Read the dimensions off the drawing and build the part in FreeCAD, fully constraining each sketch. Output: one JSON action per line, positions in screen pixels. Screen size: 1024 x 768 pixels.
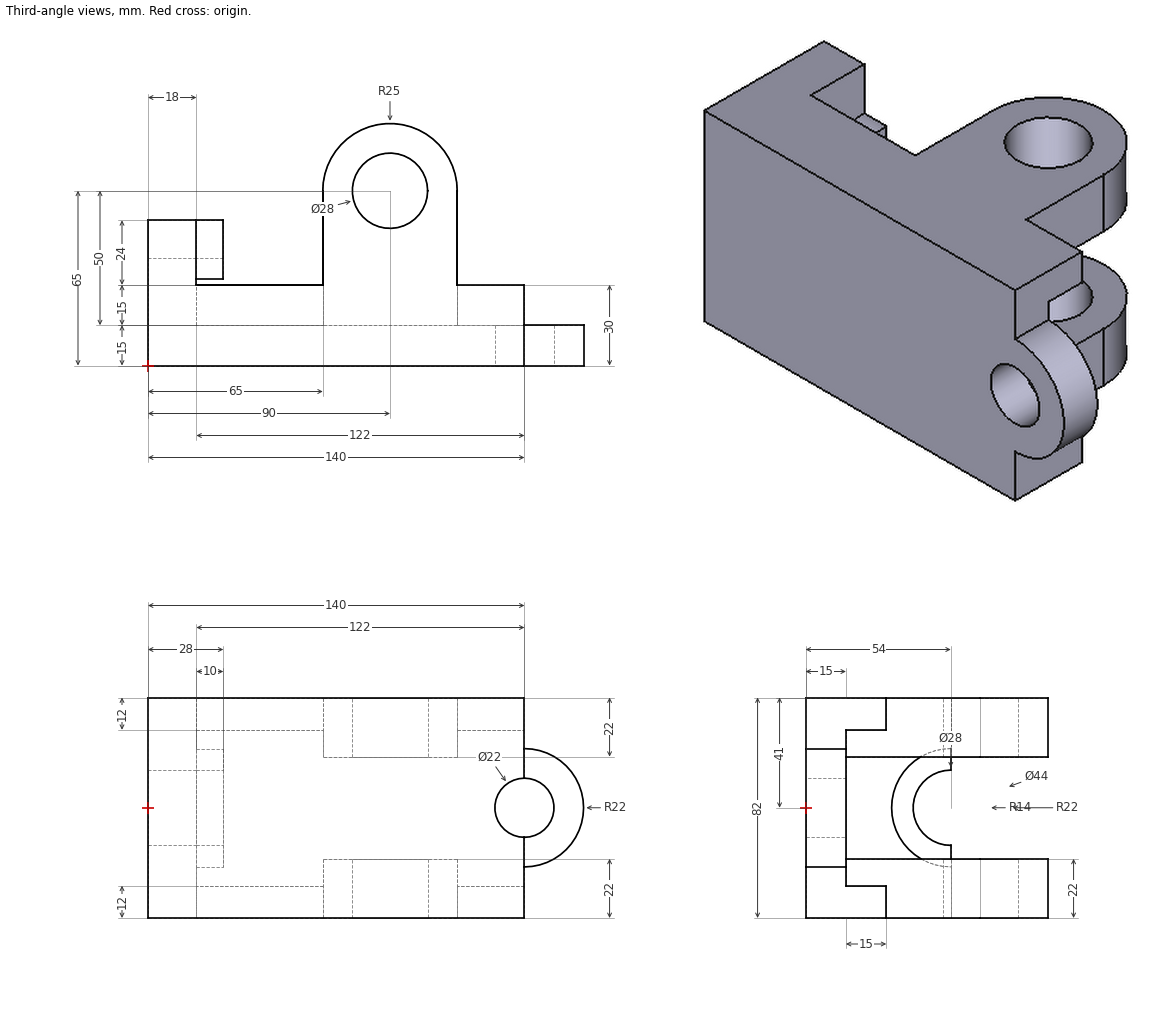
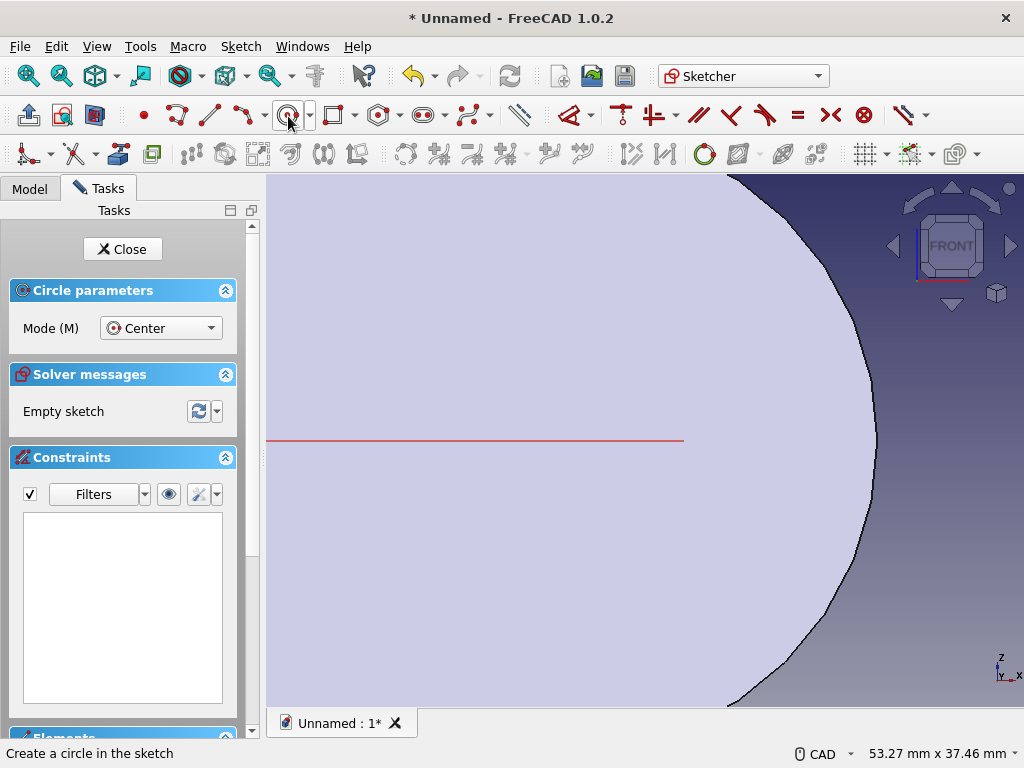
{"action": "left_click", "coordinate": [564, 440]}
{"action": "left_click", "coordinate": [675, 330]}
{"action": "key", "text": "Escape"}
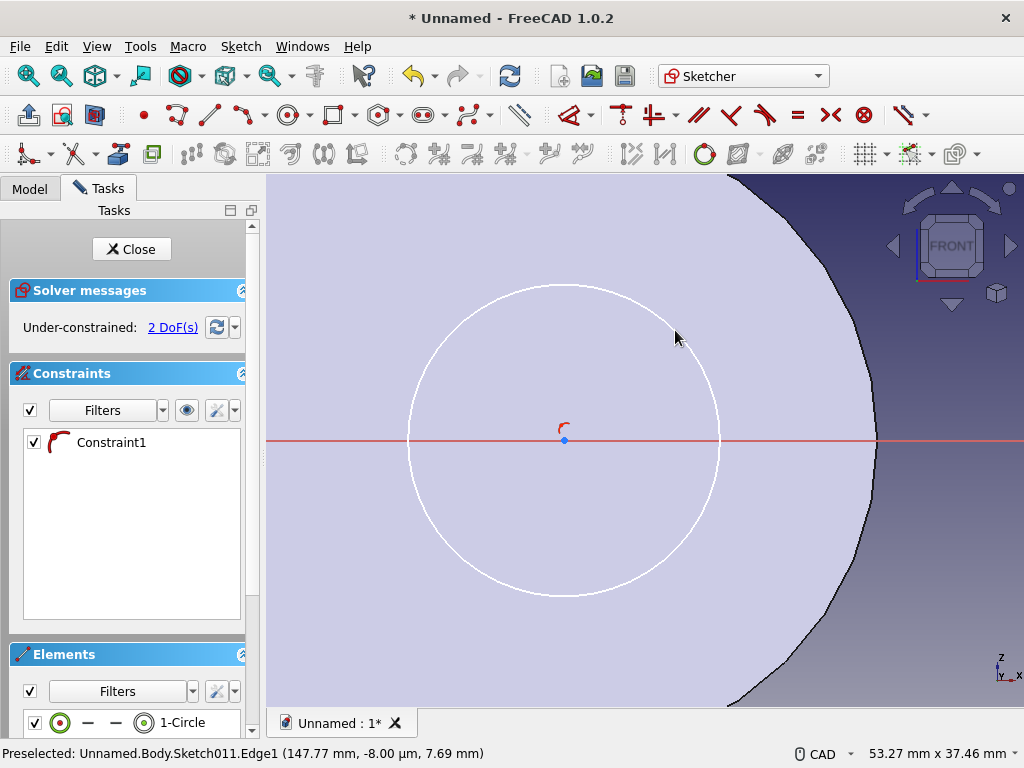
{"action": "key", "text": "d"}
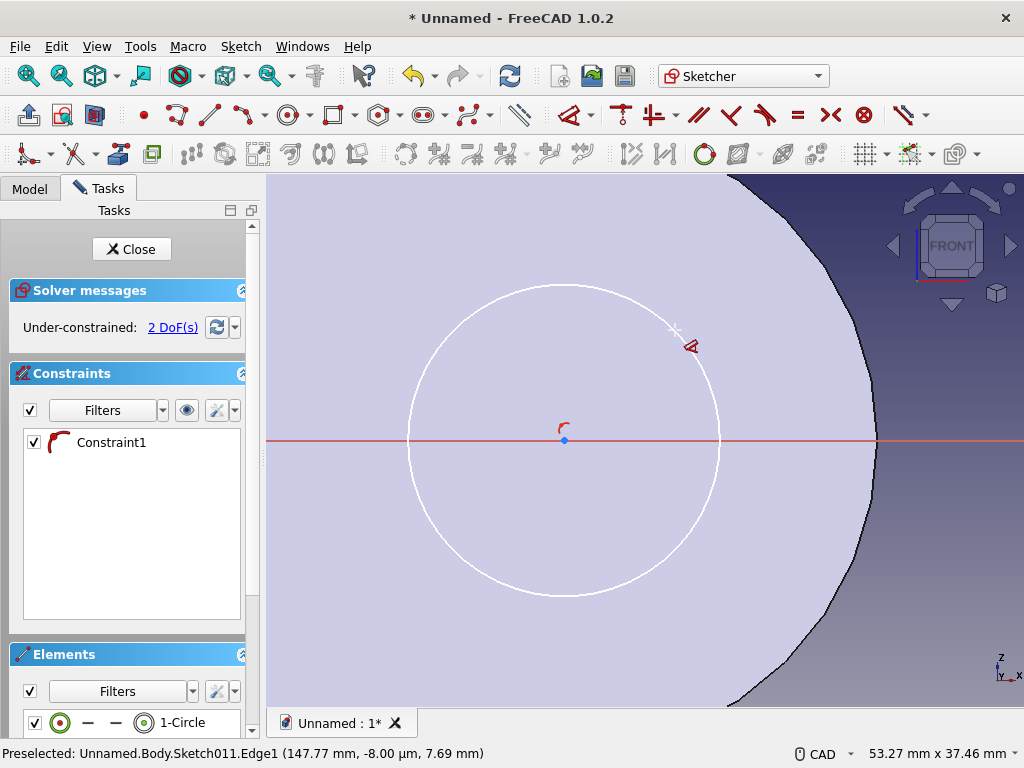
{"action": "left_click", "coordinate": [674, 330]}
{"action": "left_click", "coordinate": [697, 307]}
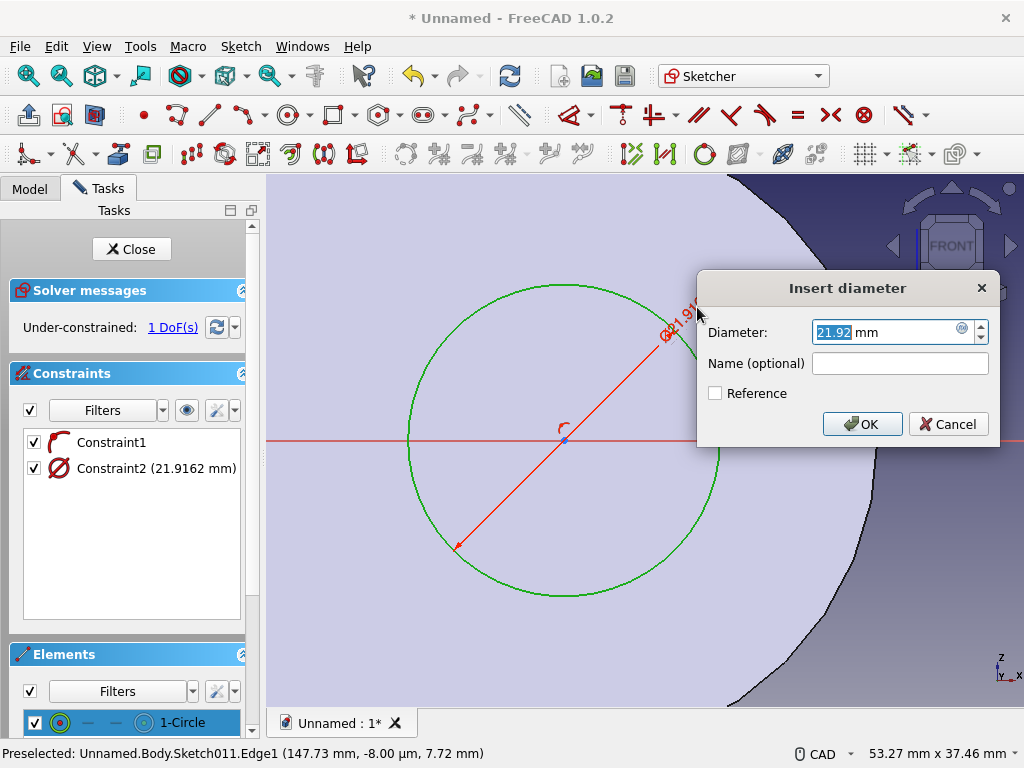
{"action": "type", "text": "22"}
{"action": "key", "text": "Return"}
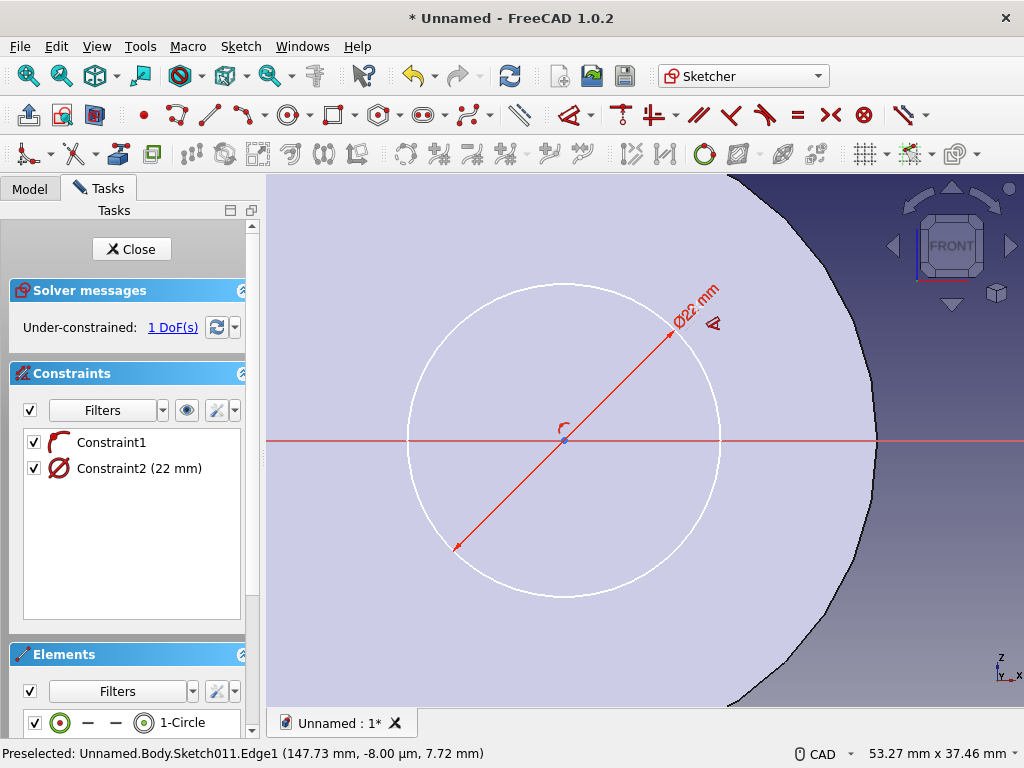
{"action": "left_click", "coordinate": [564, 440]}
{"action": "left_click", "coordinate": [429, 474]}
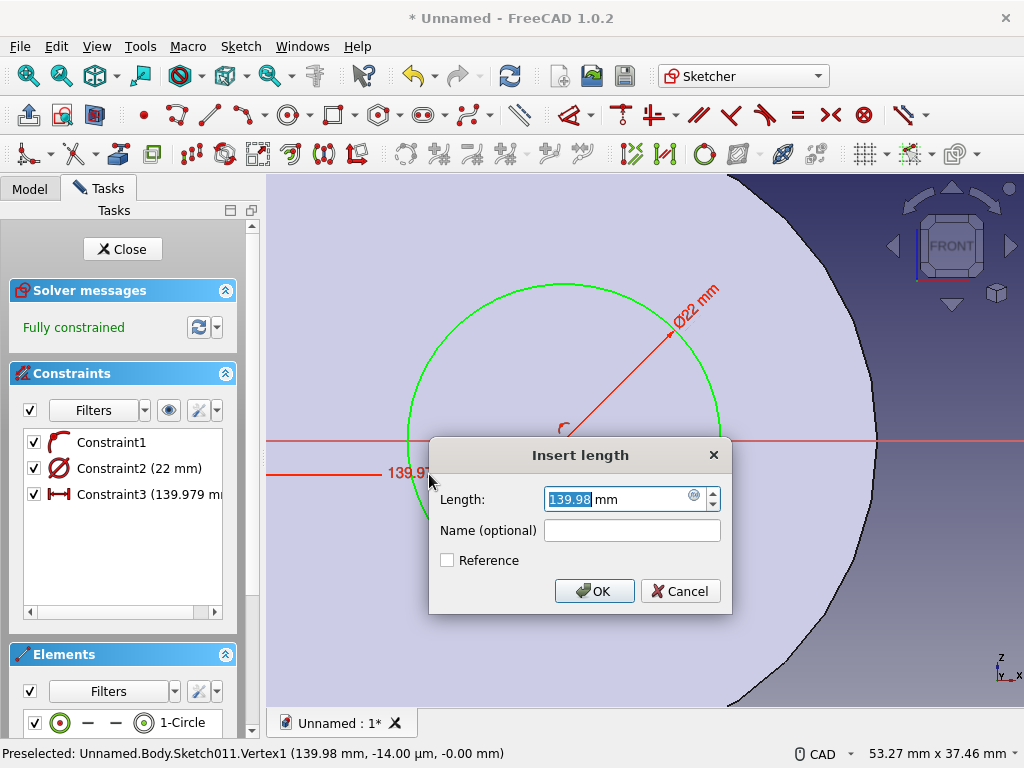
{"action": "type", "text": "140"}
{"action": "key", "text": "Return"}
{"action": "key", "text": "Escape"}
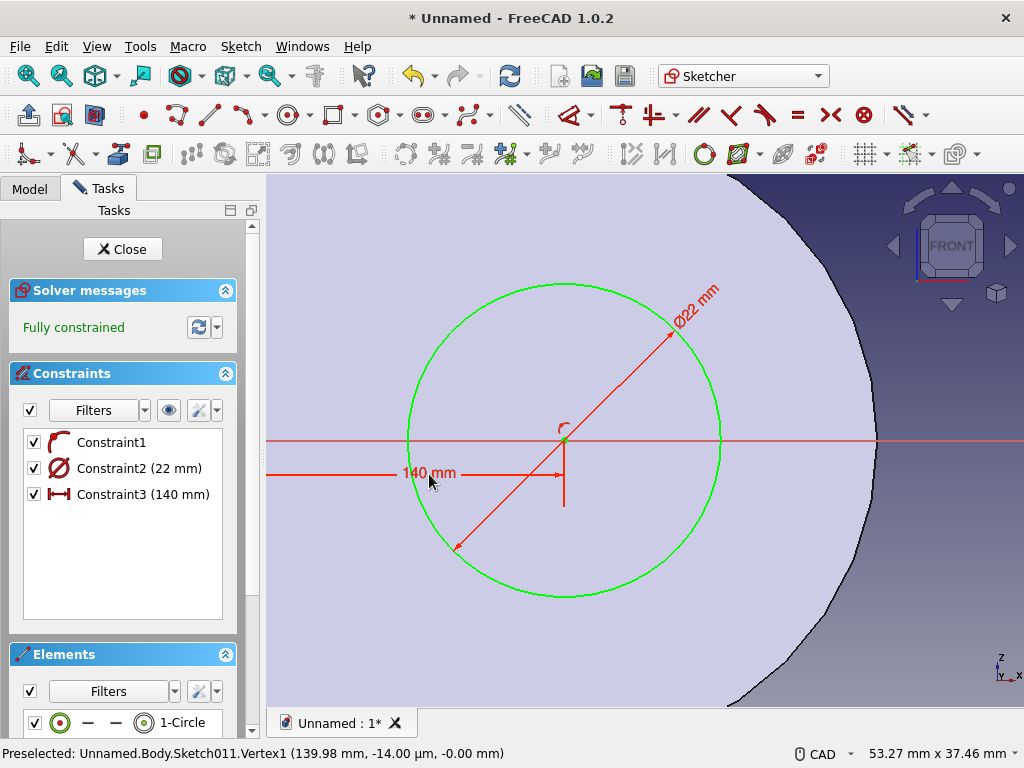
{"action": "left_click", "coordinate": [123, 249]}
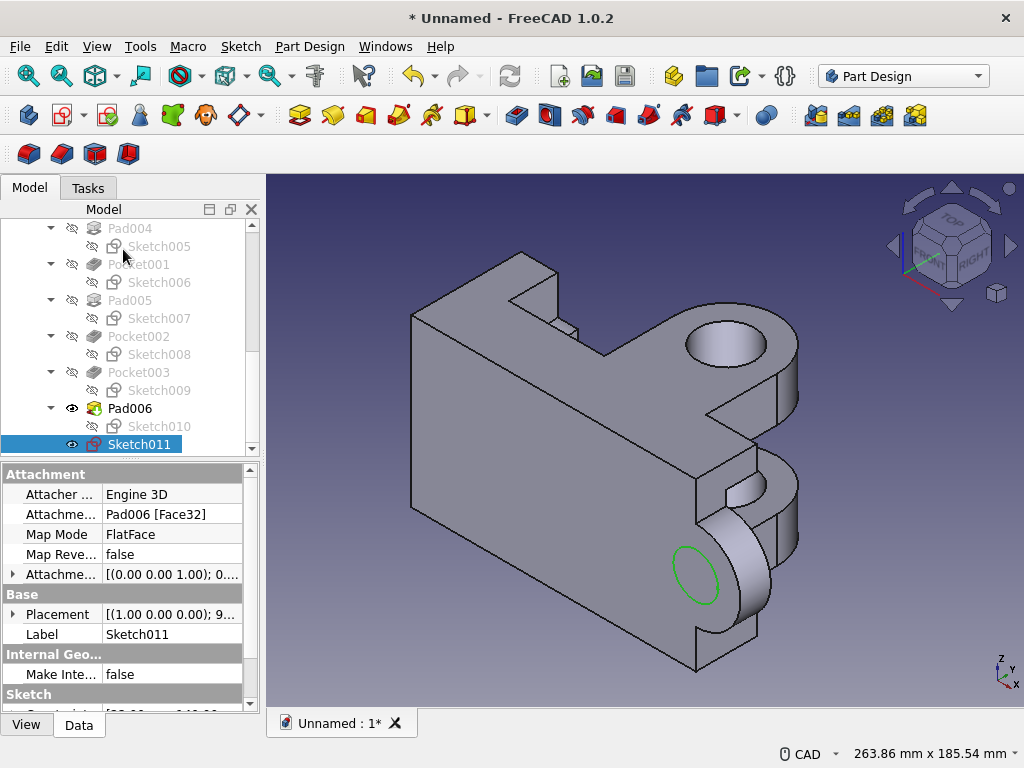
{"action": "left_click", "coordinate": [517, 116]}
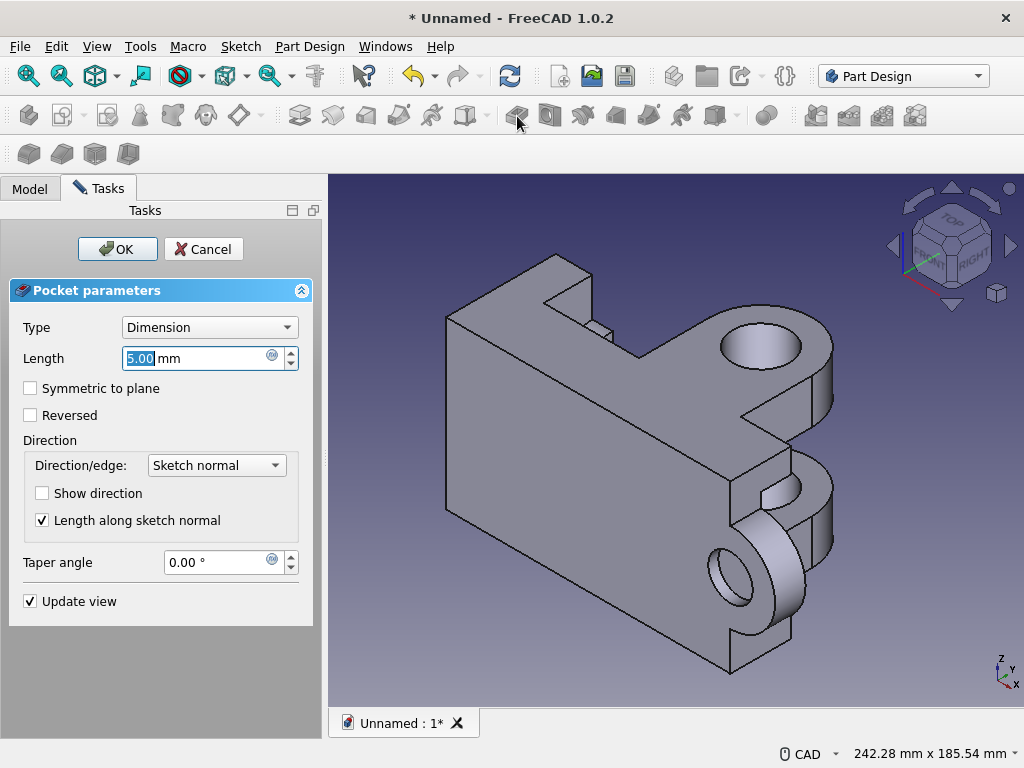
{"action": "type", "text": "15"}
{"action": "key", "text": "Tab"}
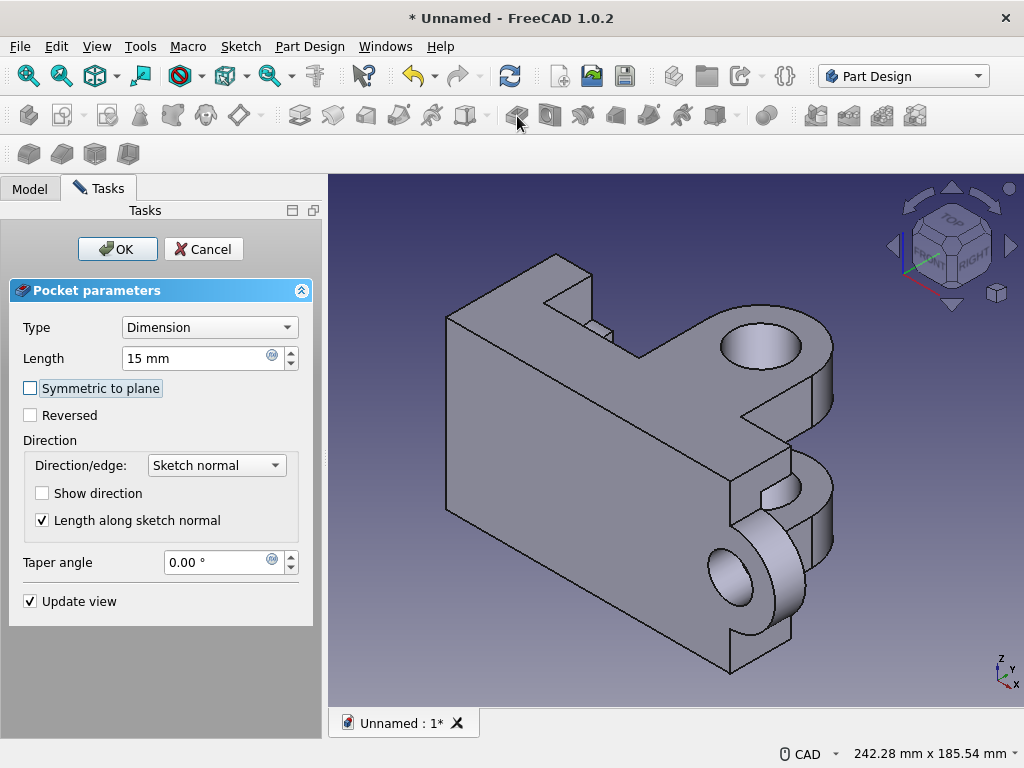
{"action": "left_click", "coordinate": [118, 249]}